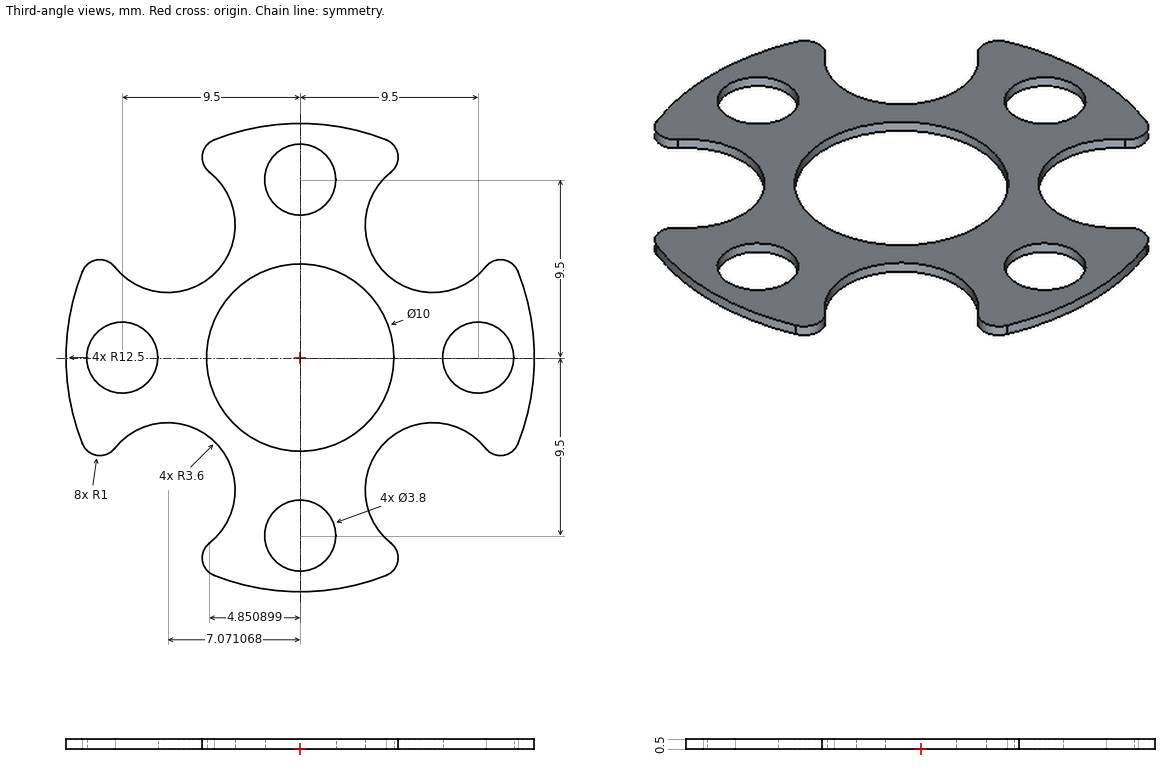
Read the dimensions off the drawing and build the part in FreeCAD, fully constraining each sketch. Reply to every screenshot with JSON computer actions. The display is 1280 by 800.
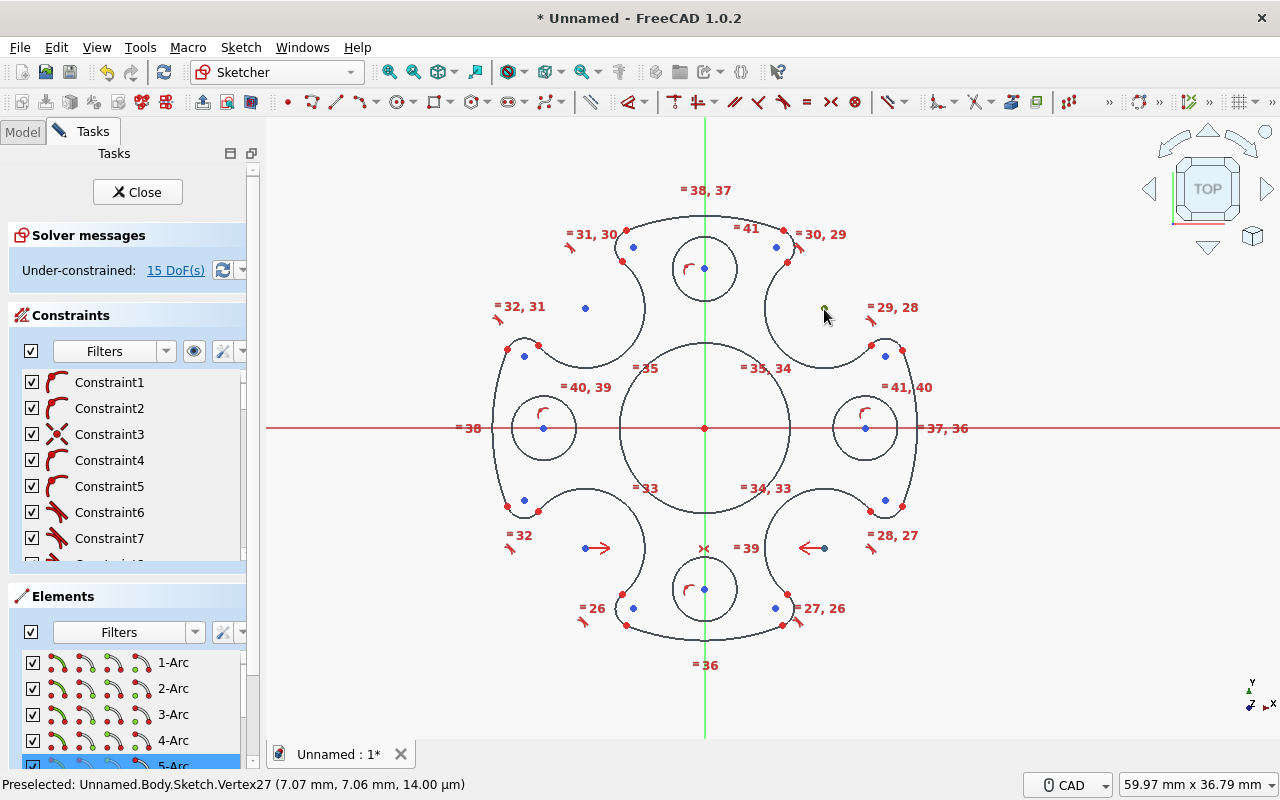
{"action": "left_click", "coordinate": [353, 428]}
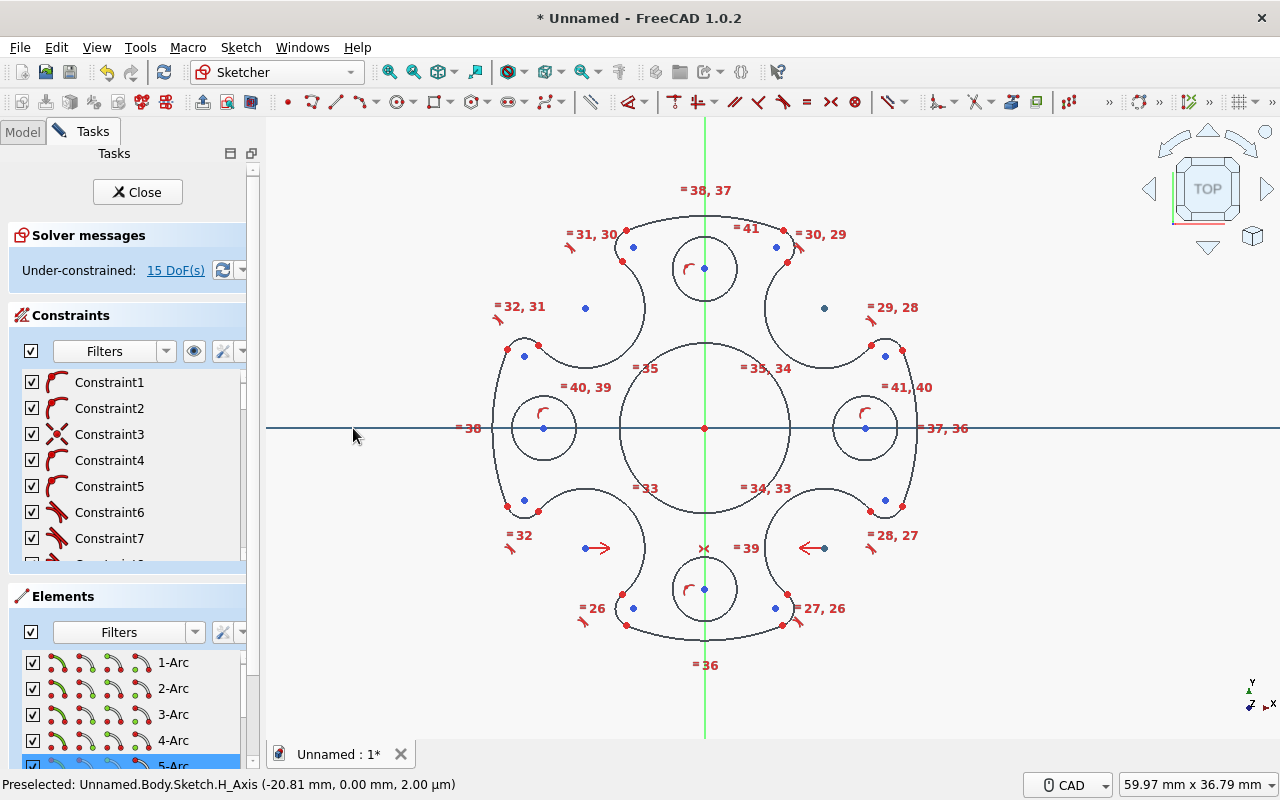
{"action": "key", "text": "s"}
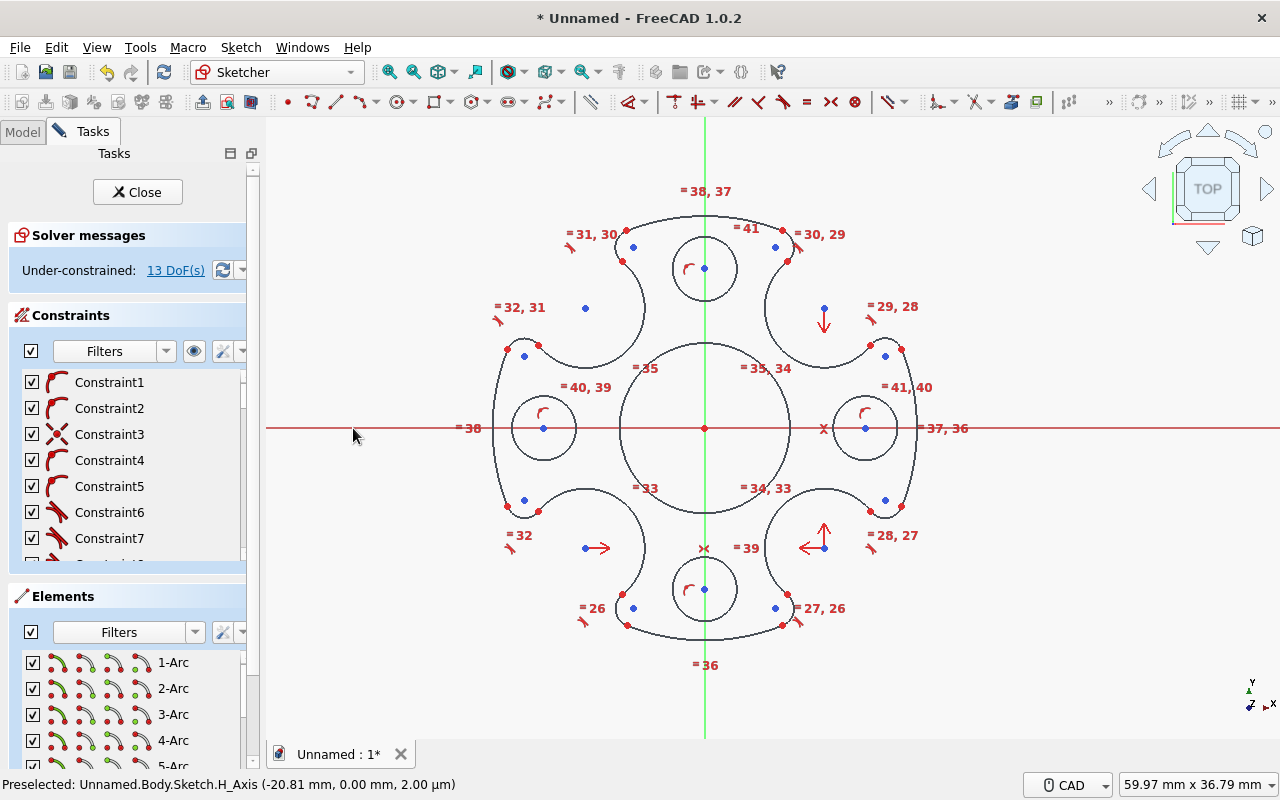
{"action": "left_click", "coordinate": [585, 548]}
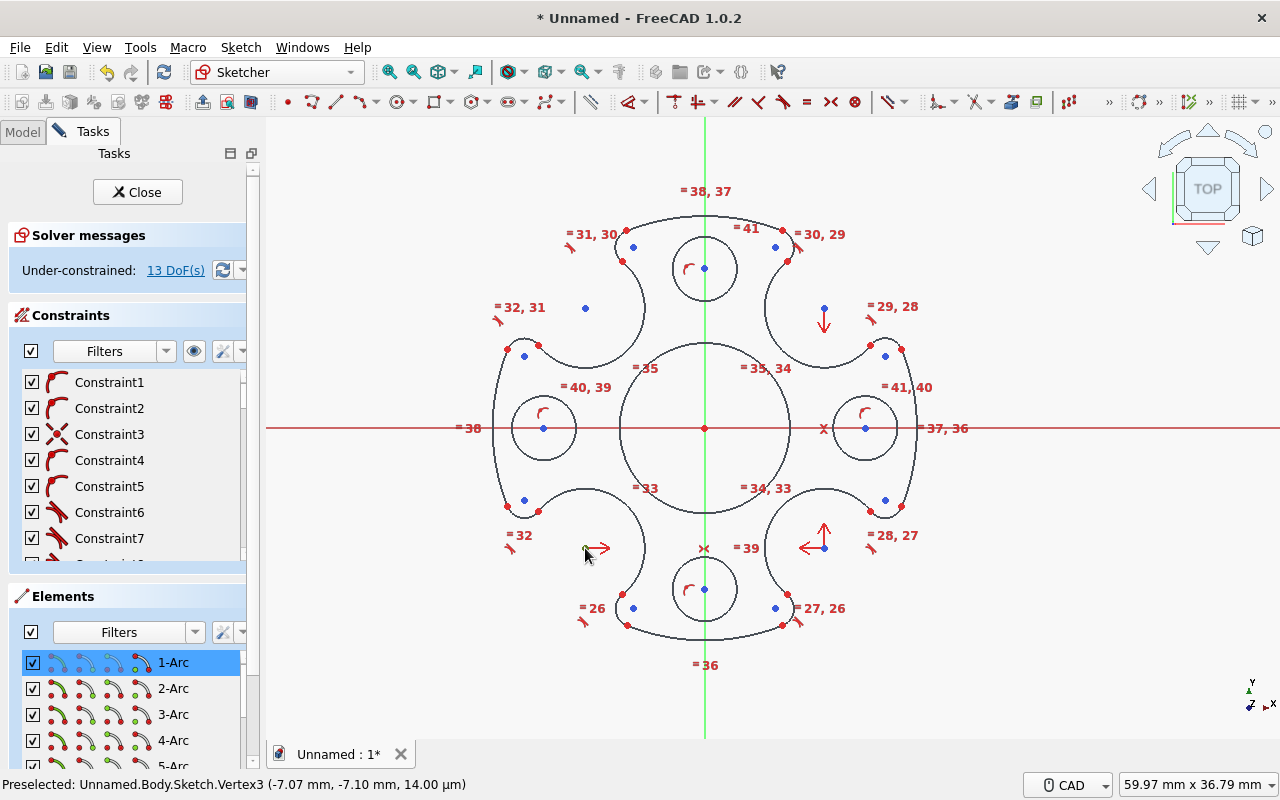
{"action": "left_click", "coordinate": [585, 309]}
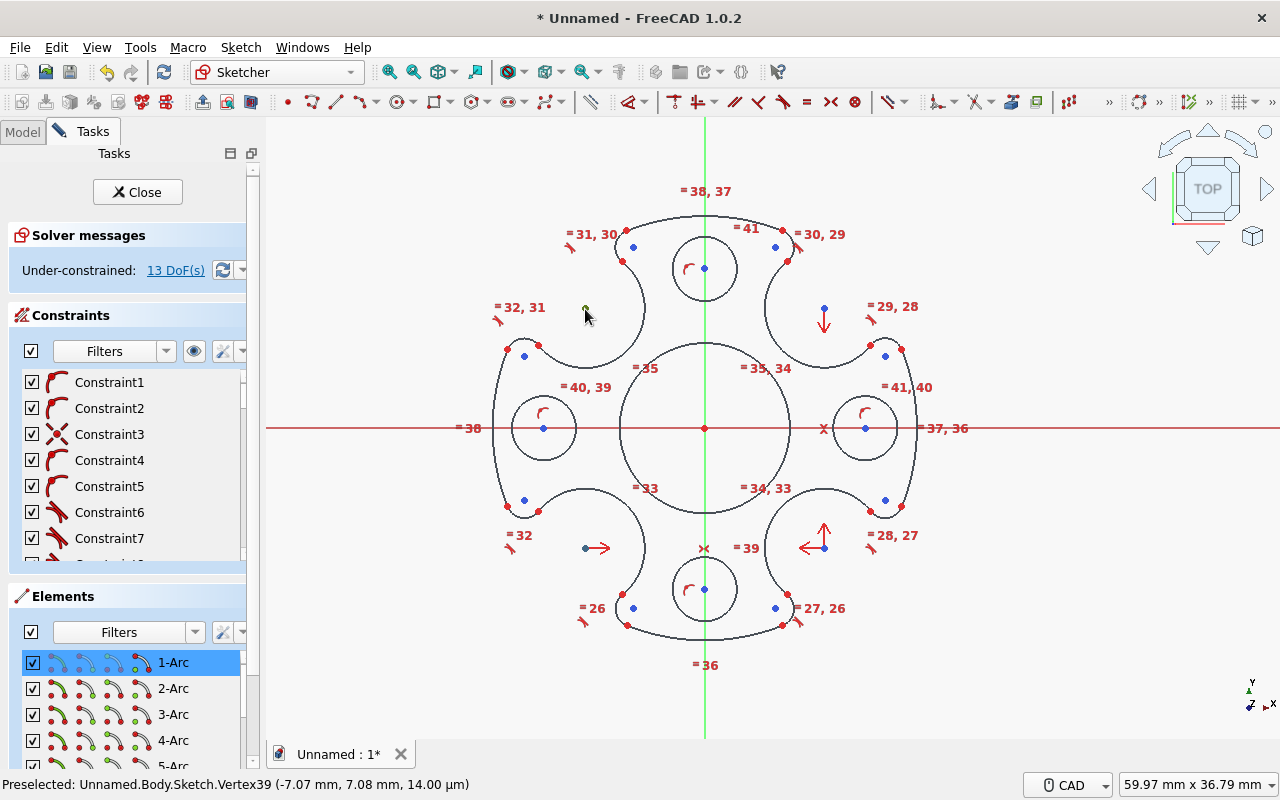
{"action": "left_click", "coordinate": [353, 428]}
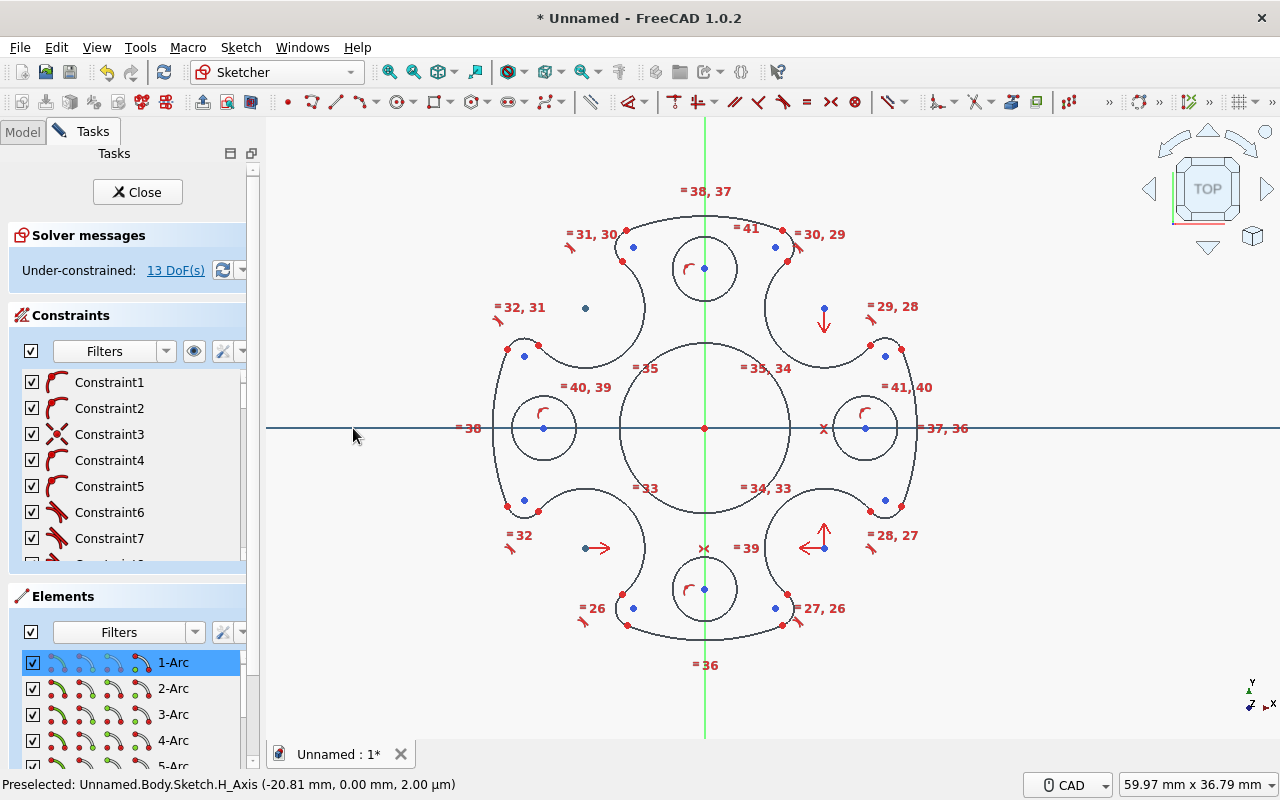
{"action": "left_click", "coordinate": [832, 102]}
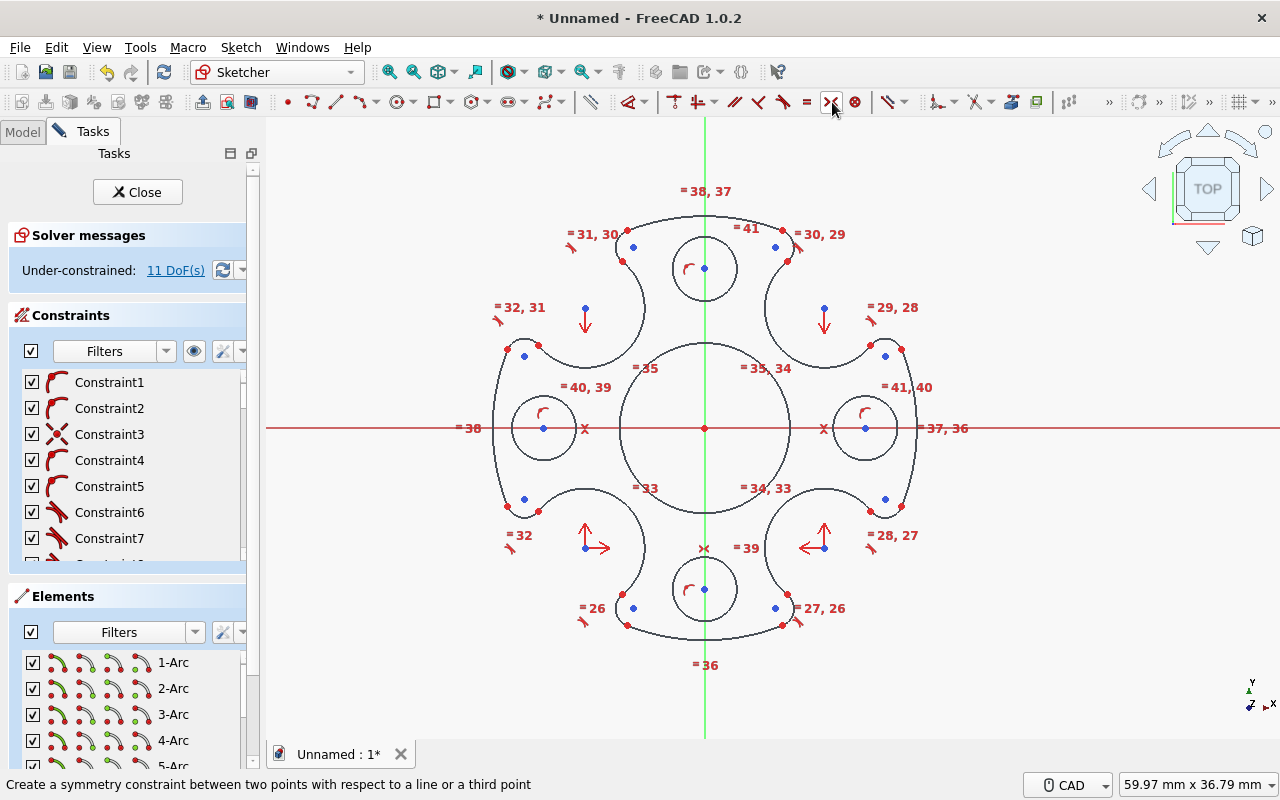
{"action": "left_click", "coordinate": [644, 541]}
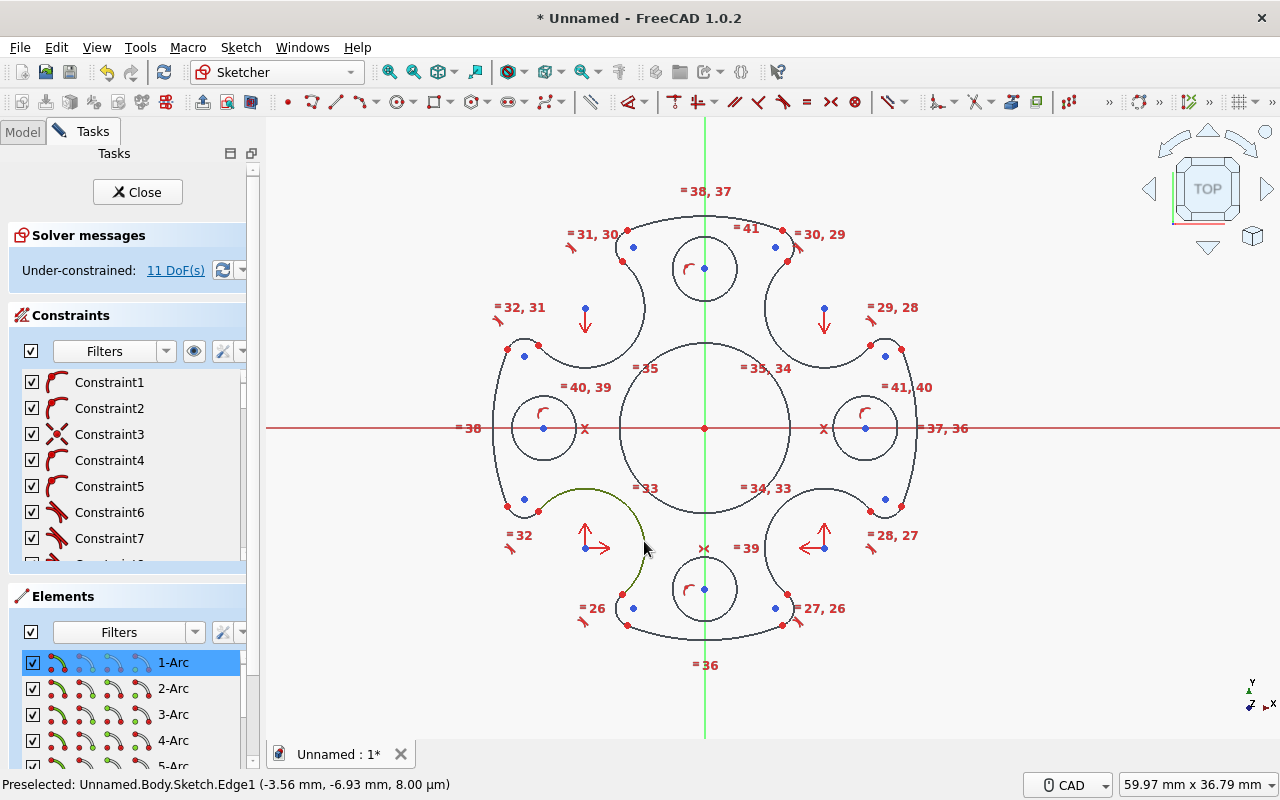
{"action": "key", "text": "k r"}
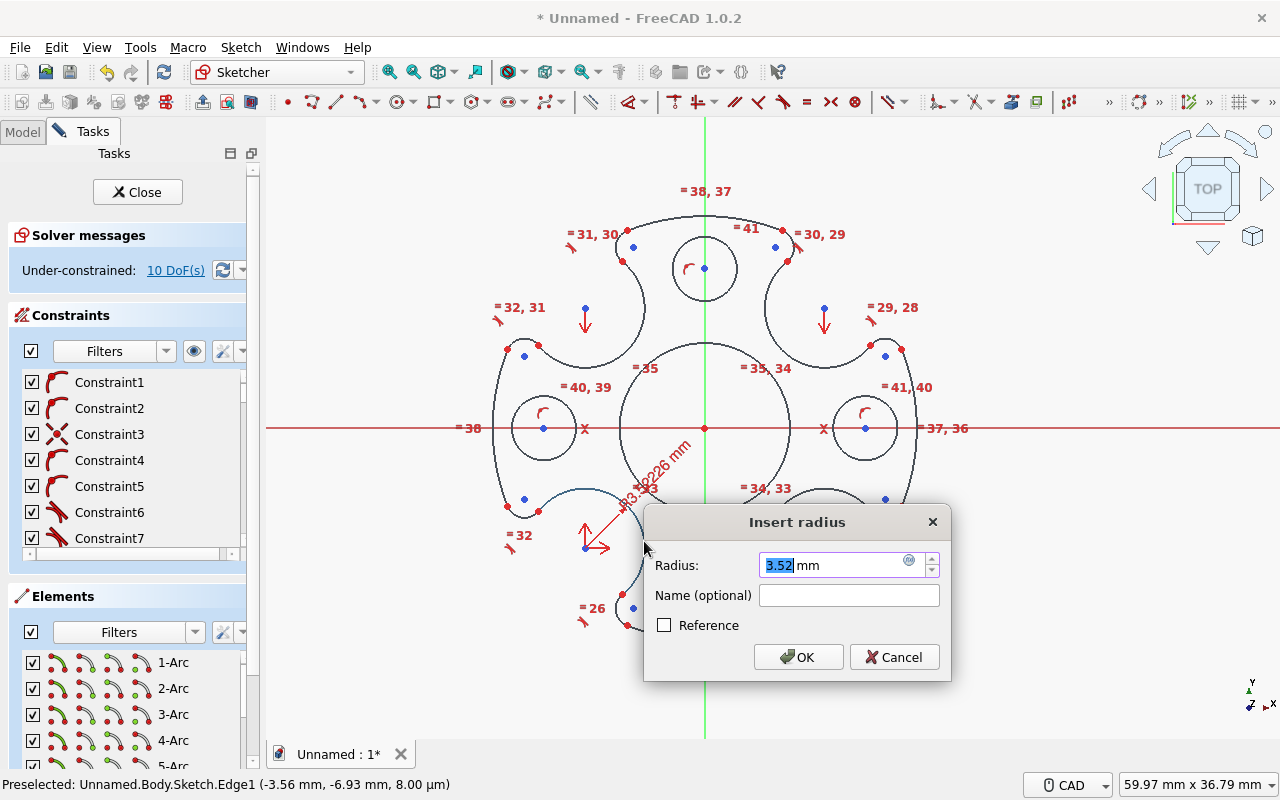
{"action": "type", "text": "3.6"}
{"action": "key", "text": "Return"}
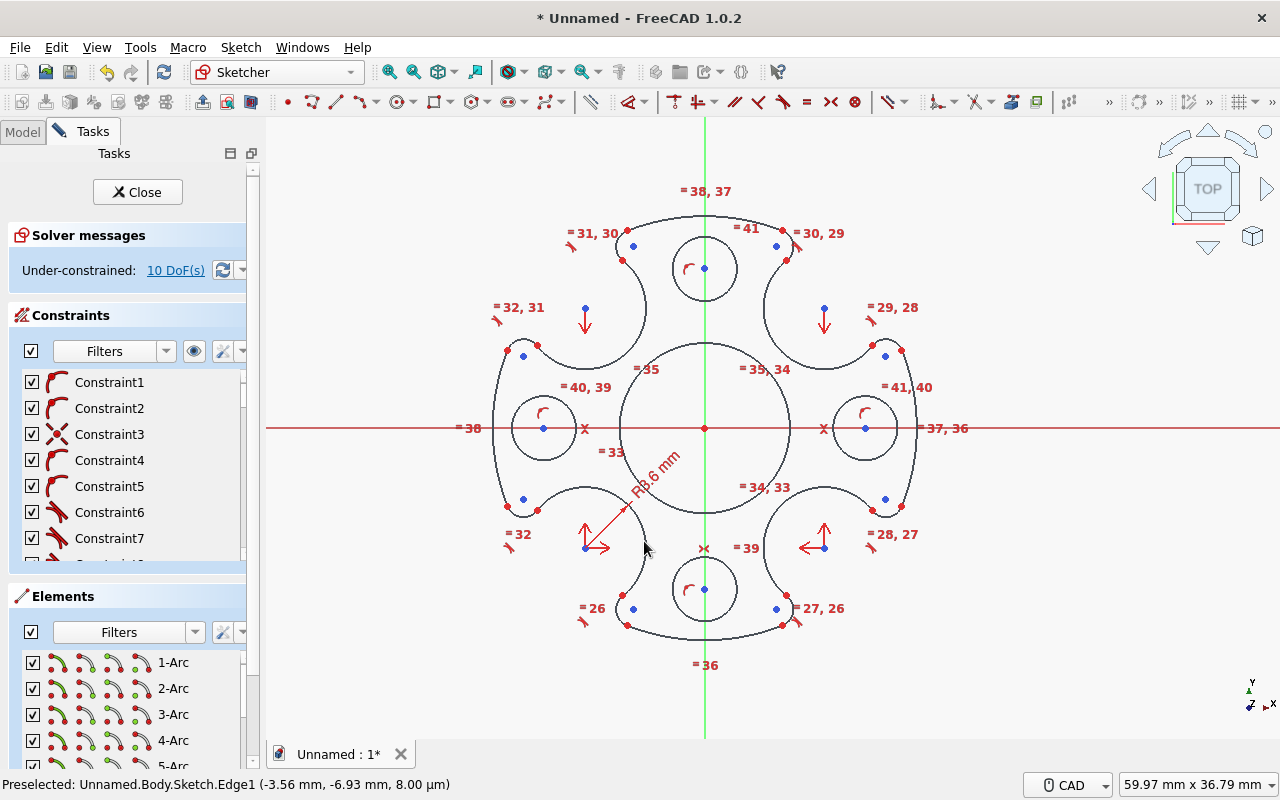
{"action": "scroll", "coordinate": [617, 605], "scroll_direction": "up", "scroll_amount": 5}